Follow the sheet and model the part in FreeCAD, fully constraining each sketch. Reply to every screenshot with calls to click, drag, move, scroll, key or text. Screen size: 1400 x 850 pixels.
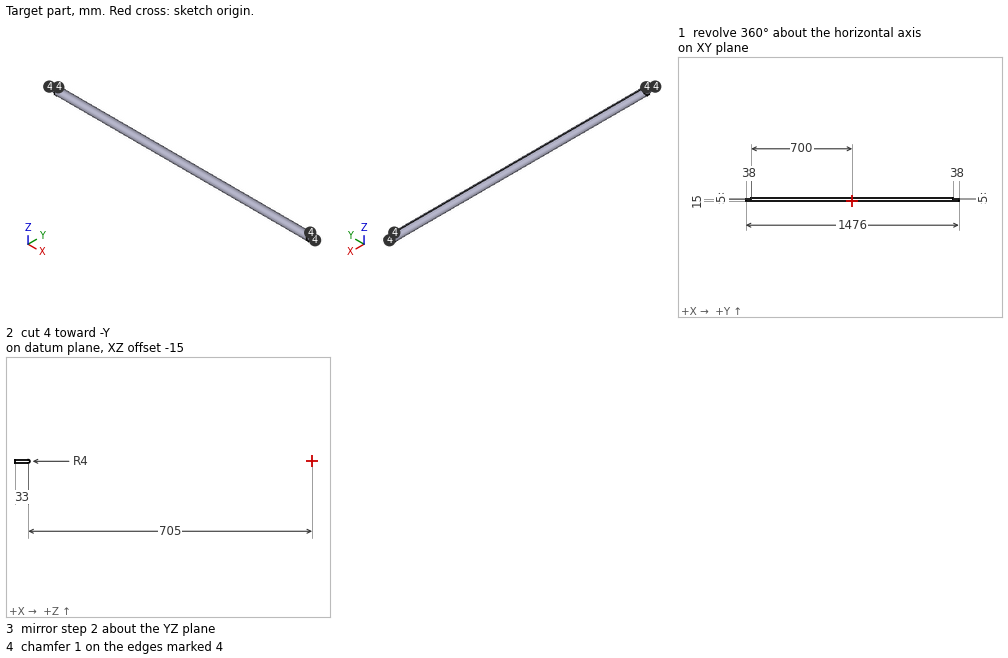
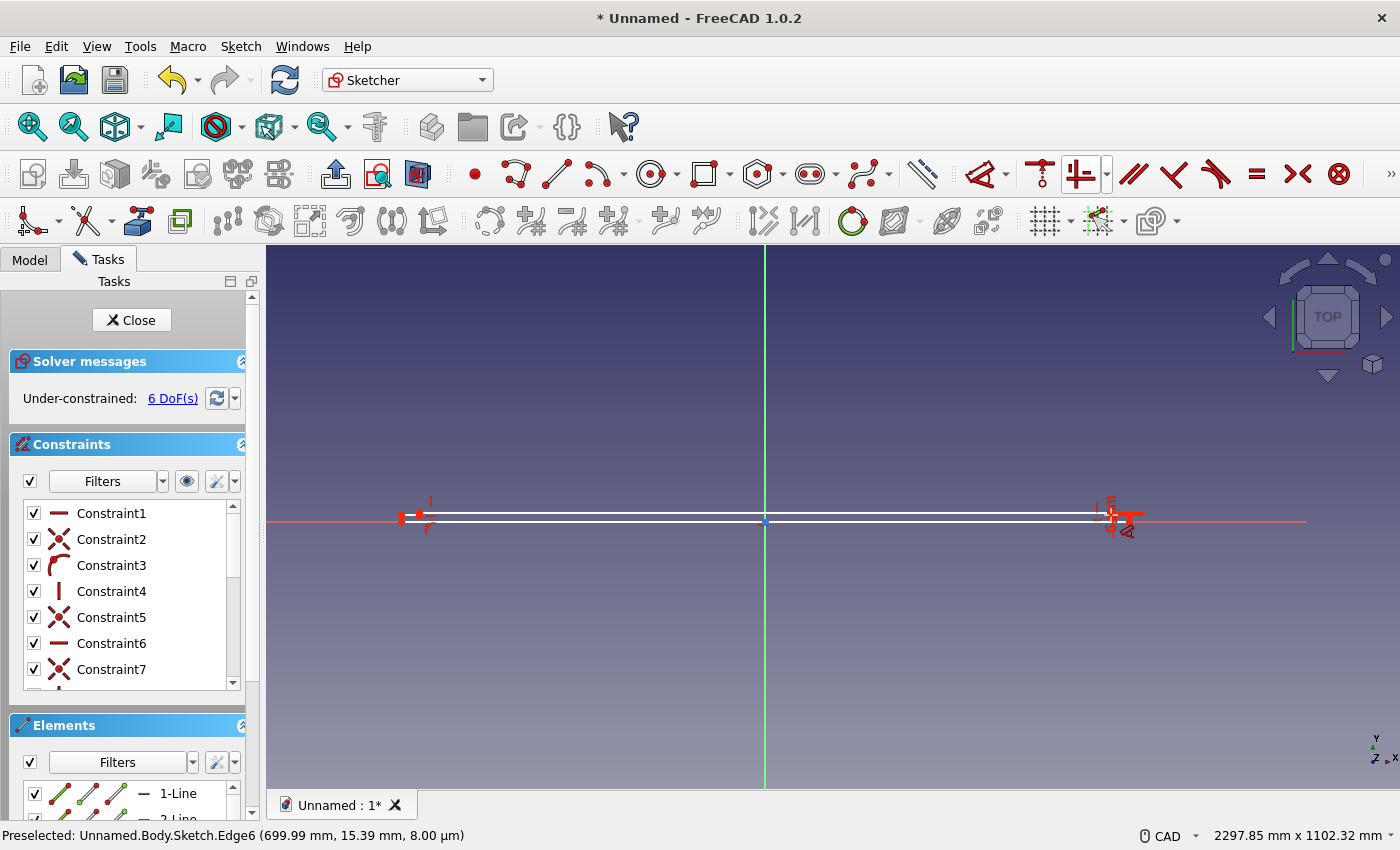
scroll(420, 513, up, 14)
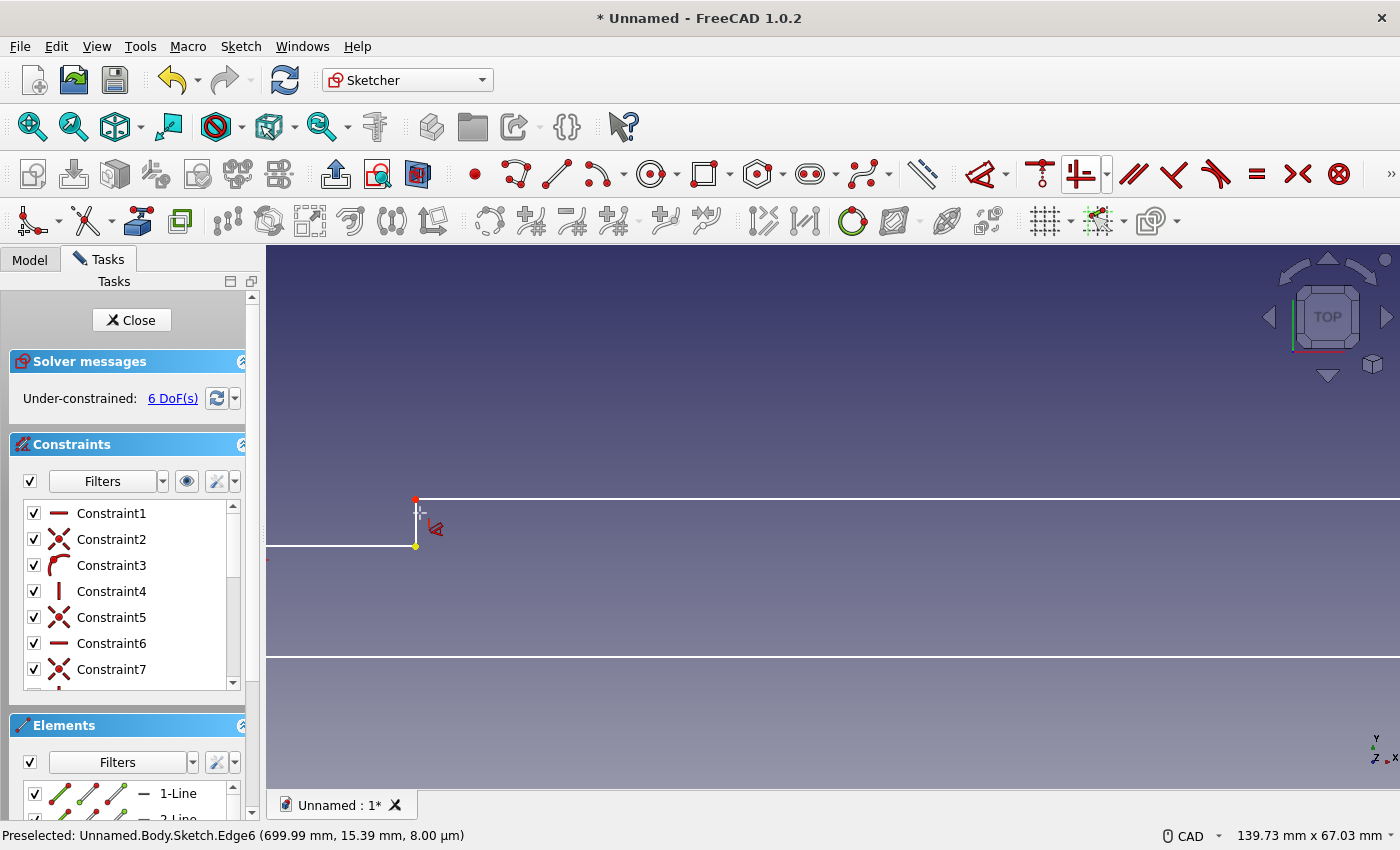
click(416, 513)
click(382, 523)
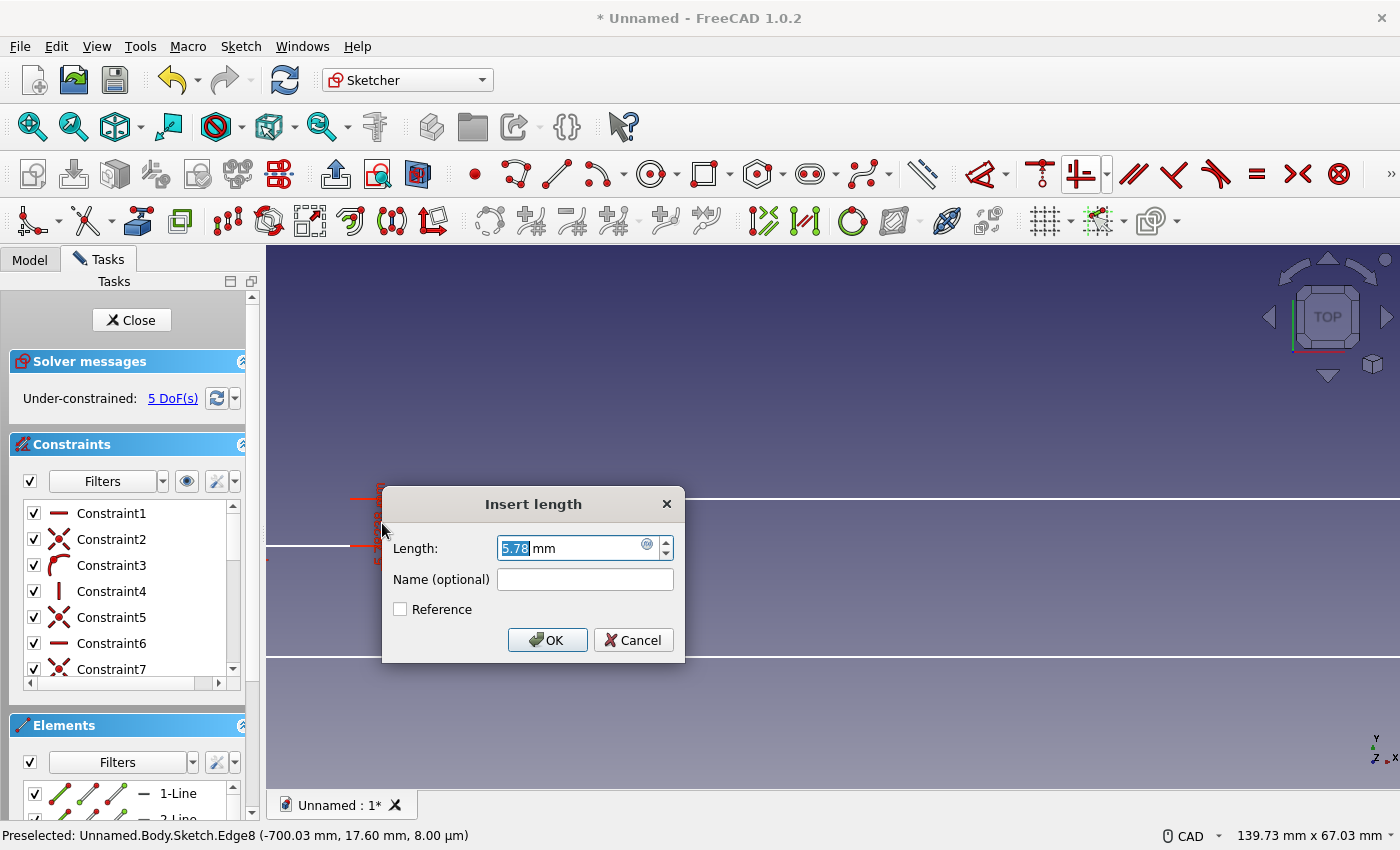
text(5)
key(Return)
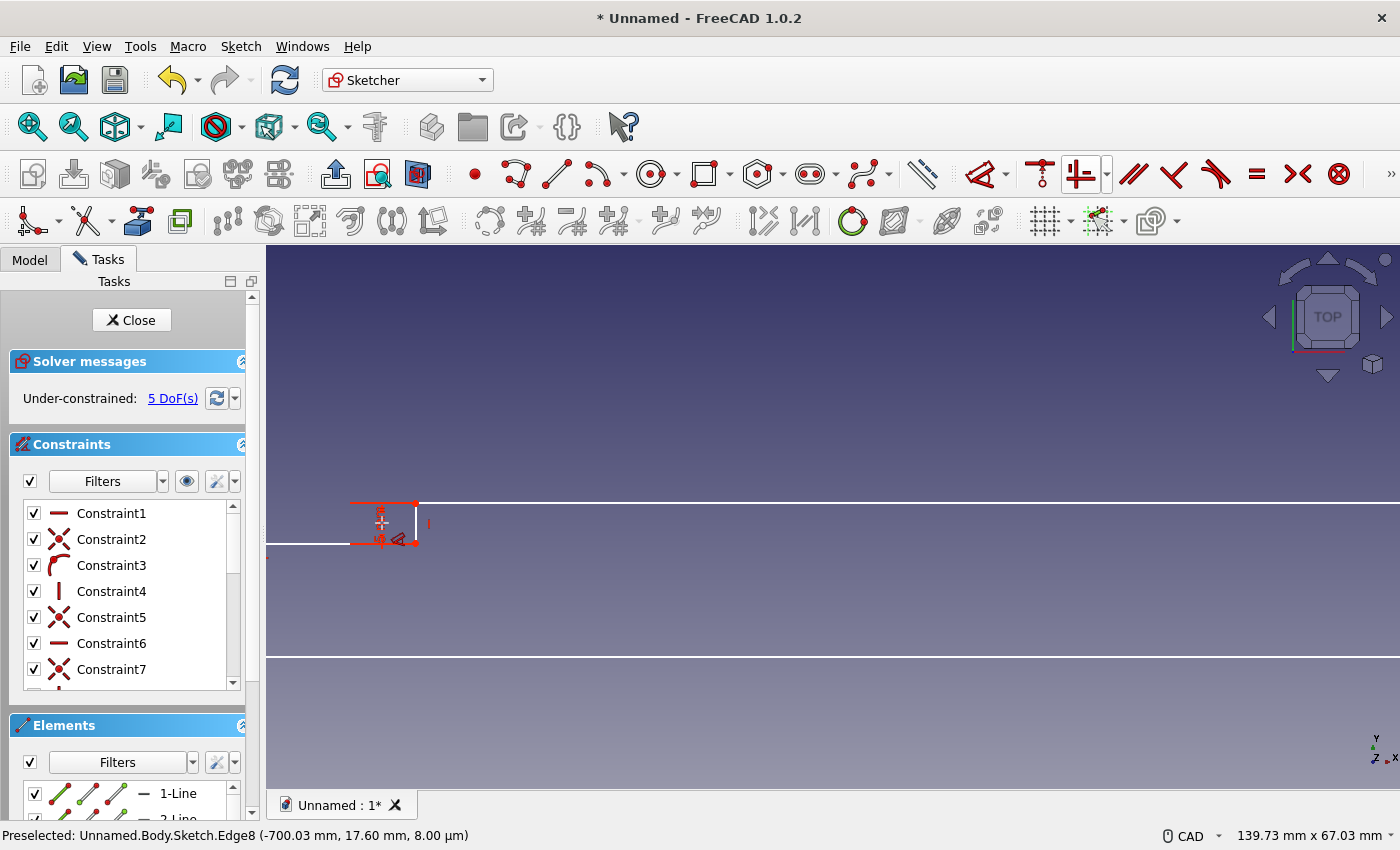
scroll(419, 513, down, 14)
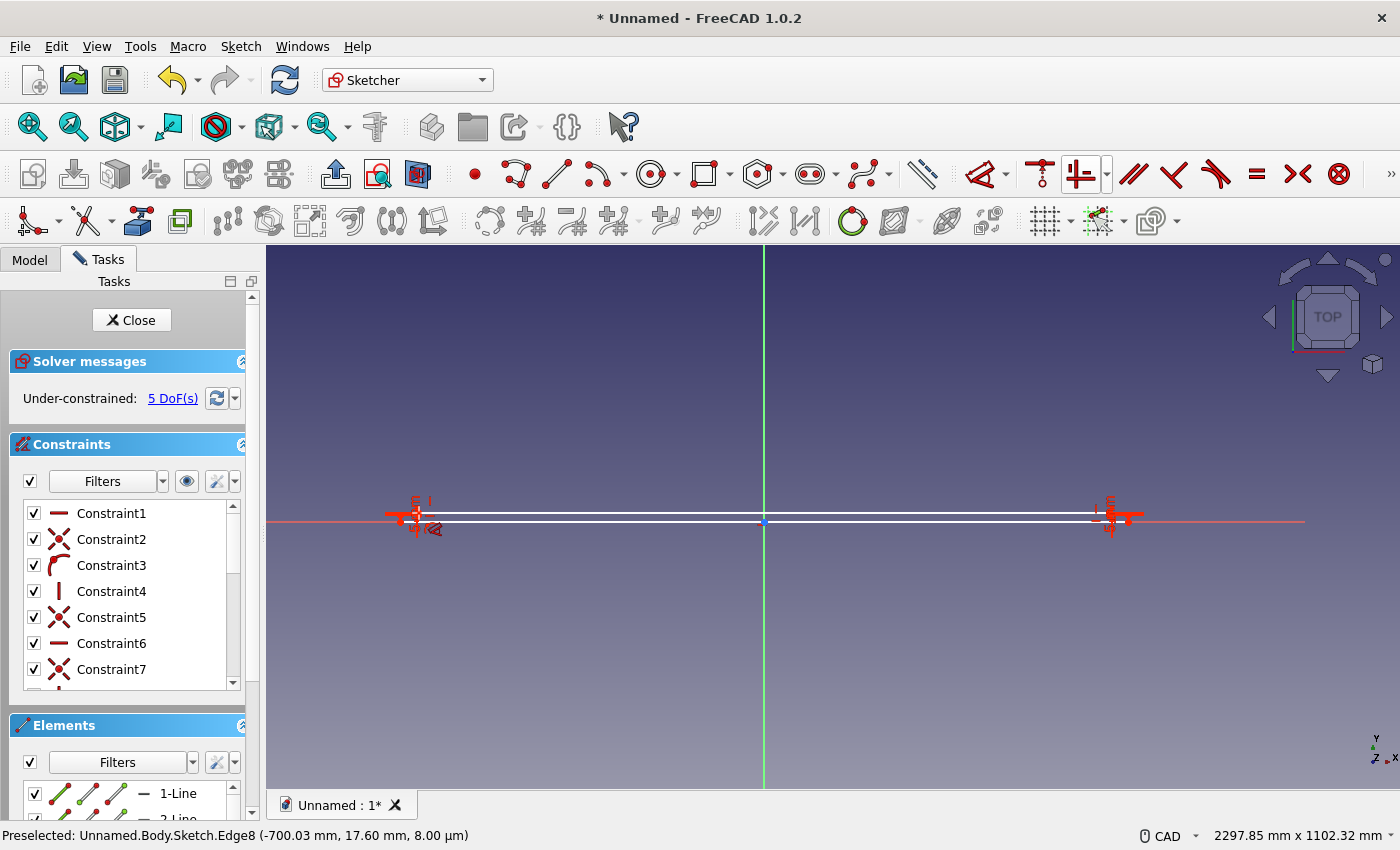
scroll(413, 515, up, 5)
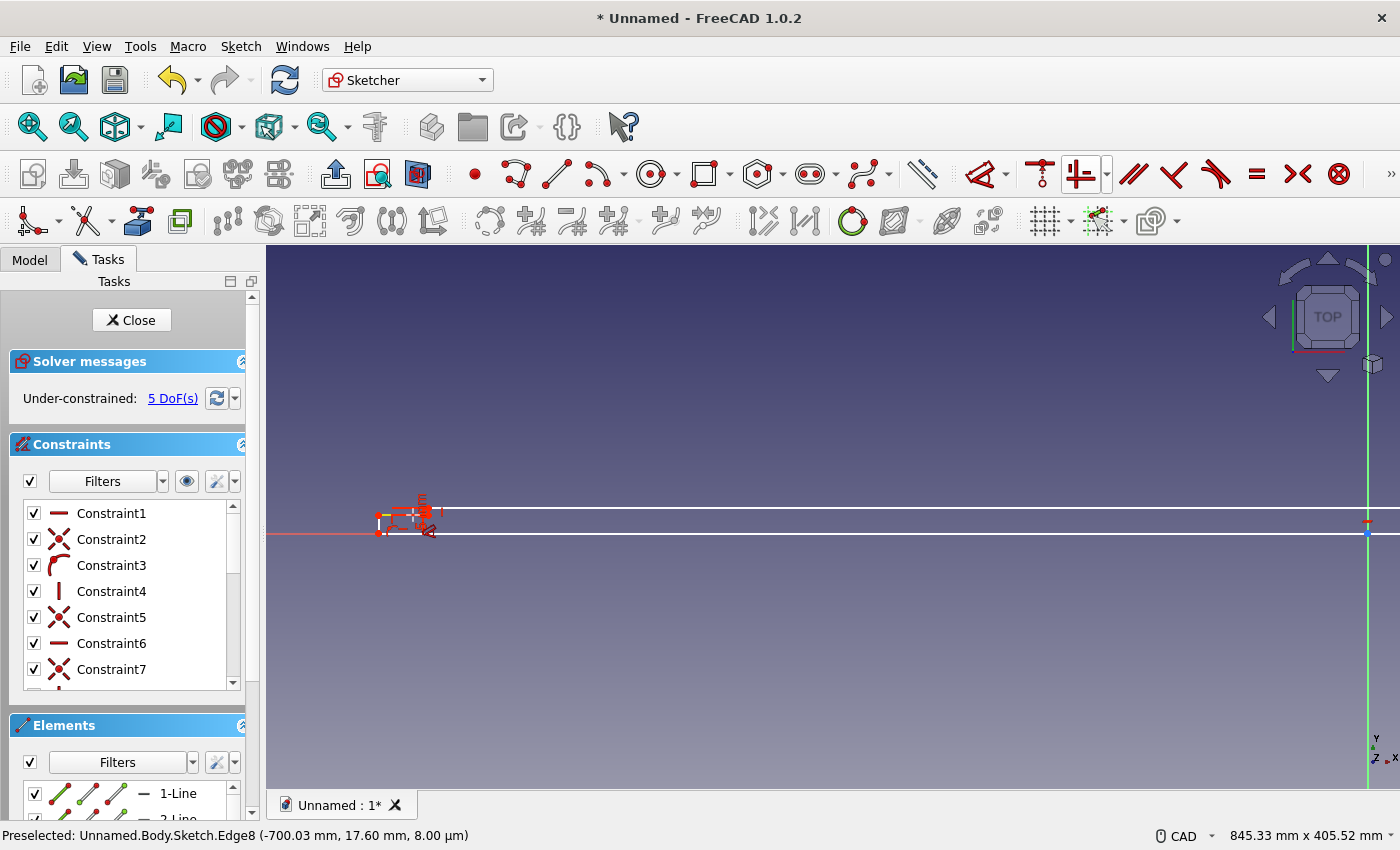
click(414, 515)
click(404, 481)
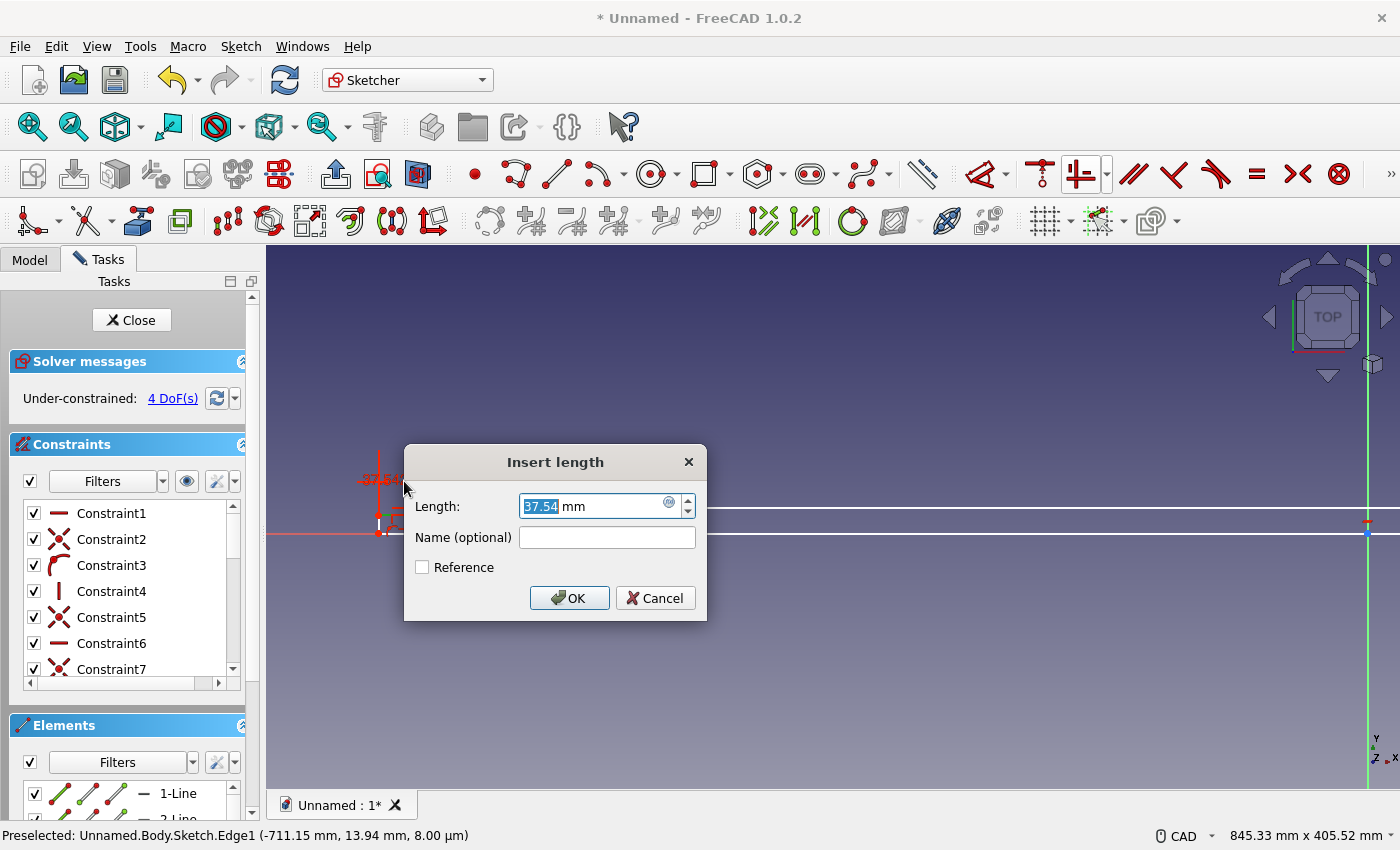
text(38)
key(Return)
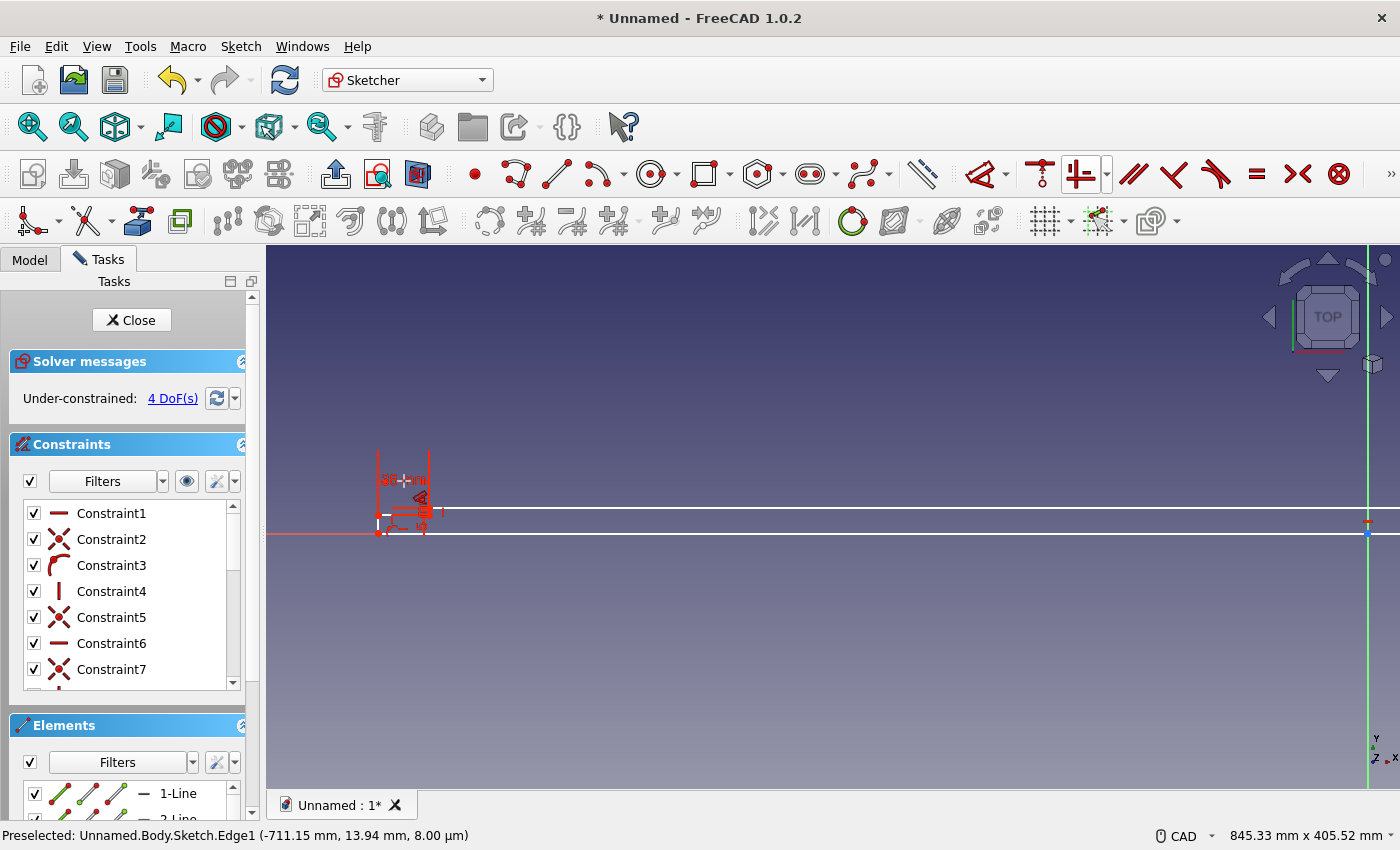
scroll(378, 524, up, 4)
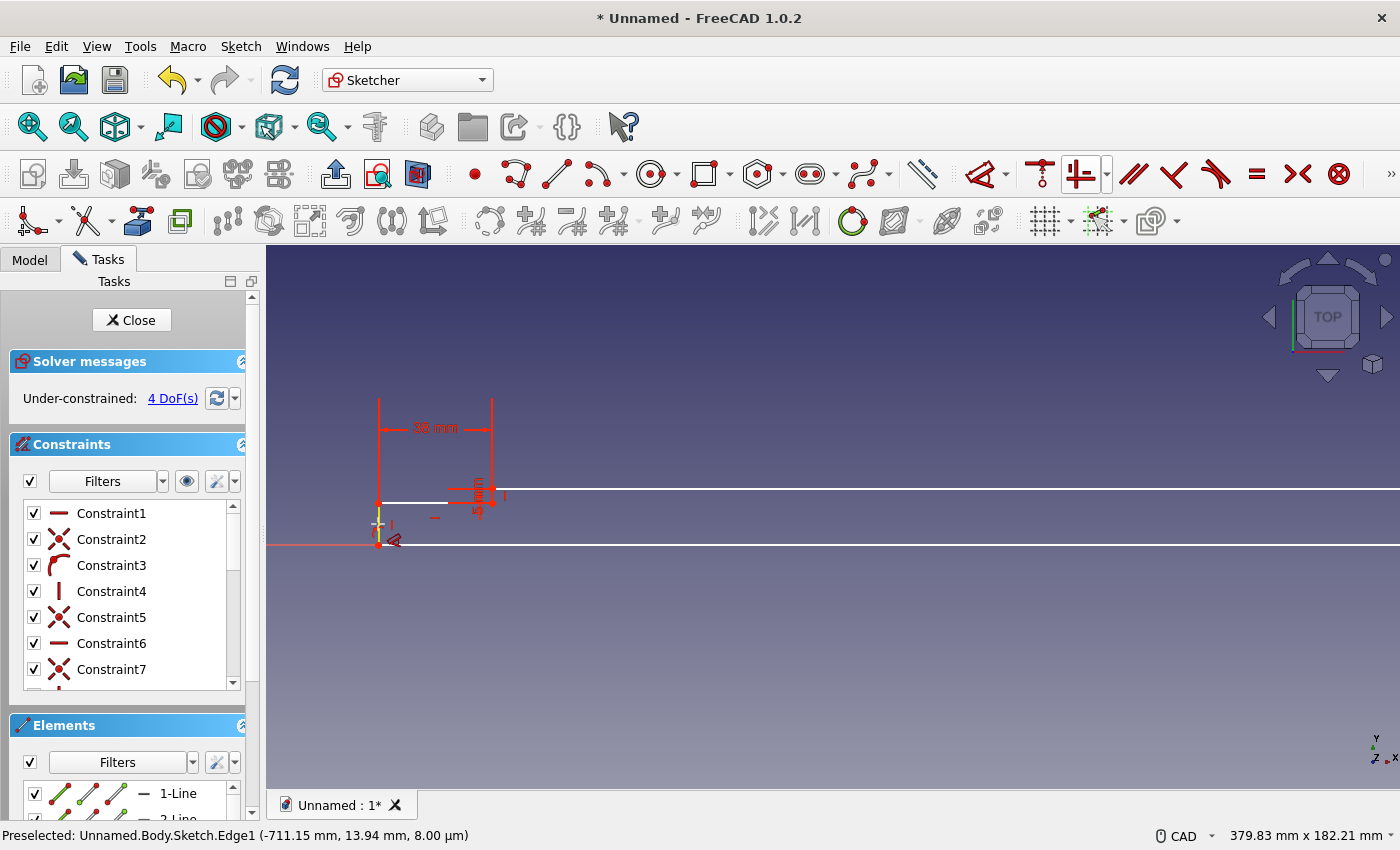
click(379, 524)
click(345, 524)